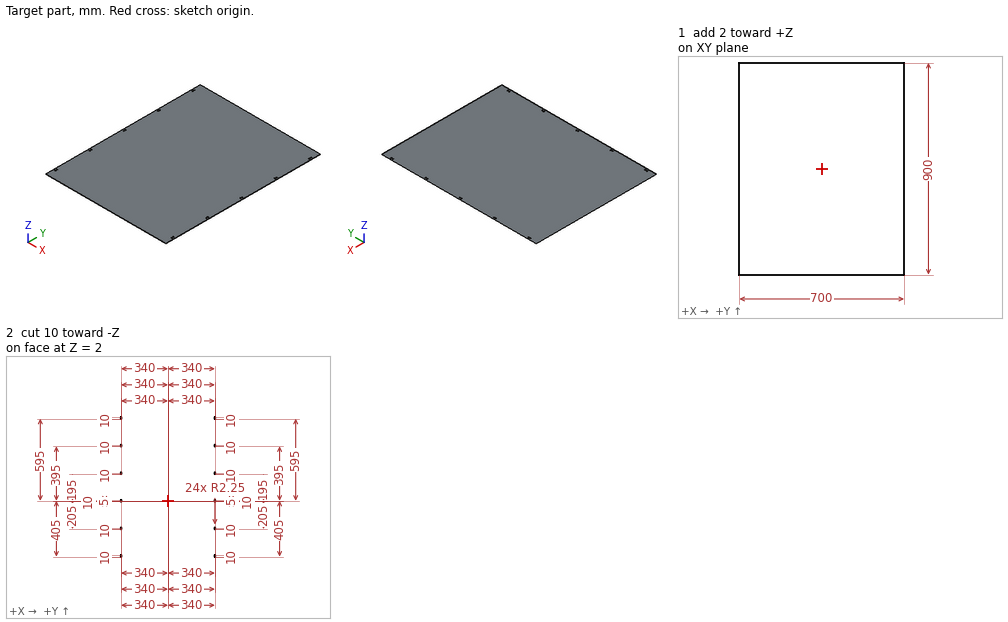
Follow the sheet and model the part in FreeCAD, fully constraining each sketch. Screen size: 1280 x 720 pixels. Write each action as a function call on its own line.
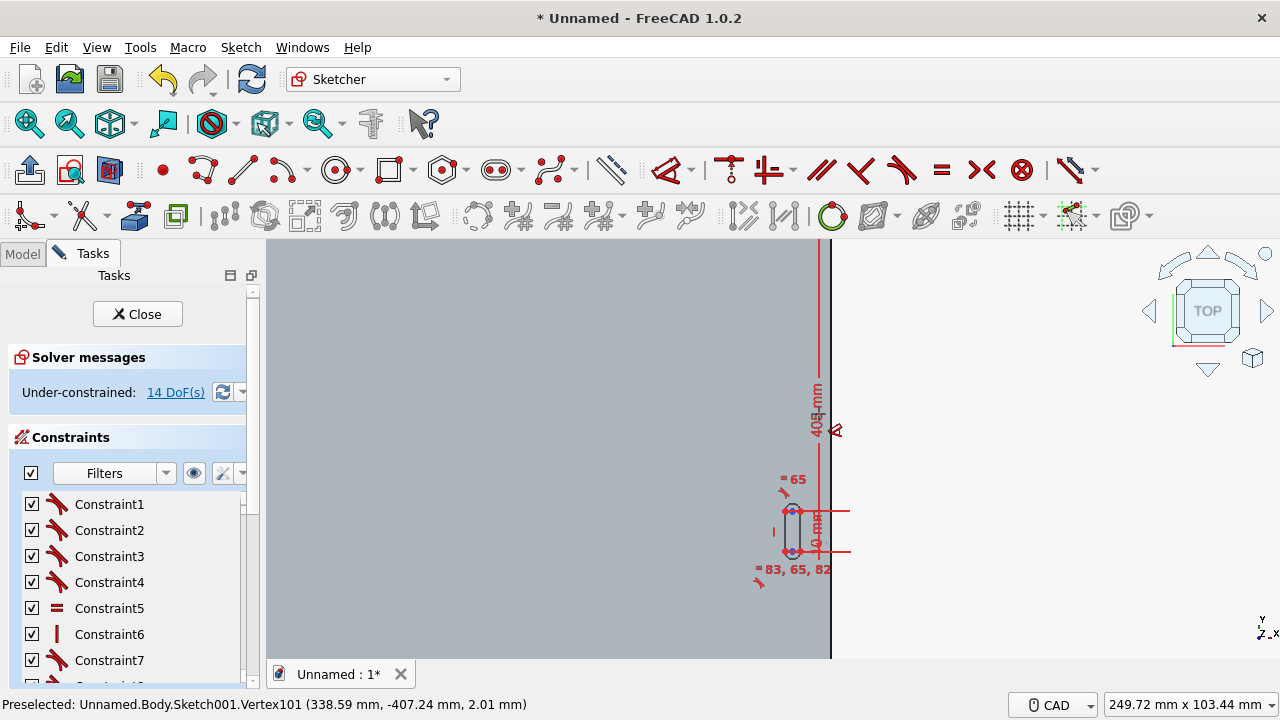
scroll(788, 575, down, 14)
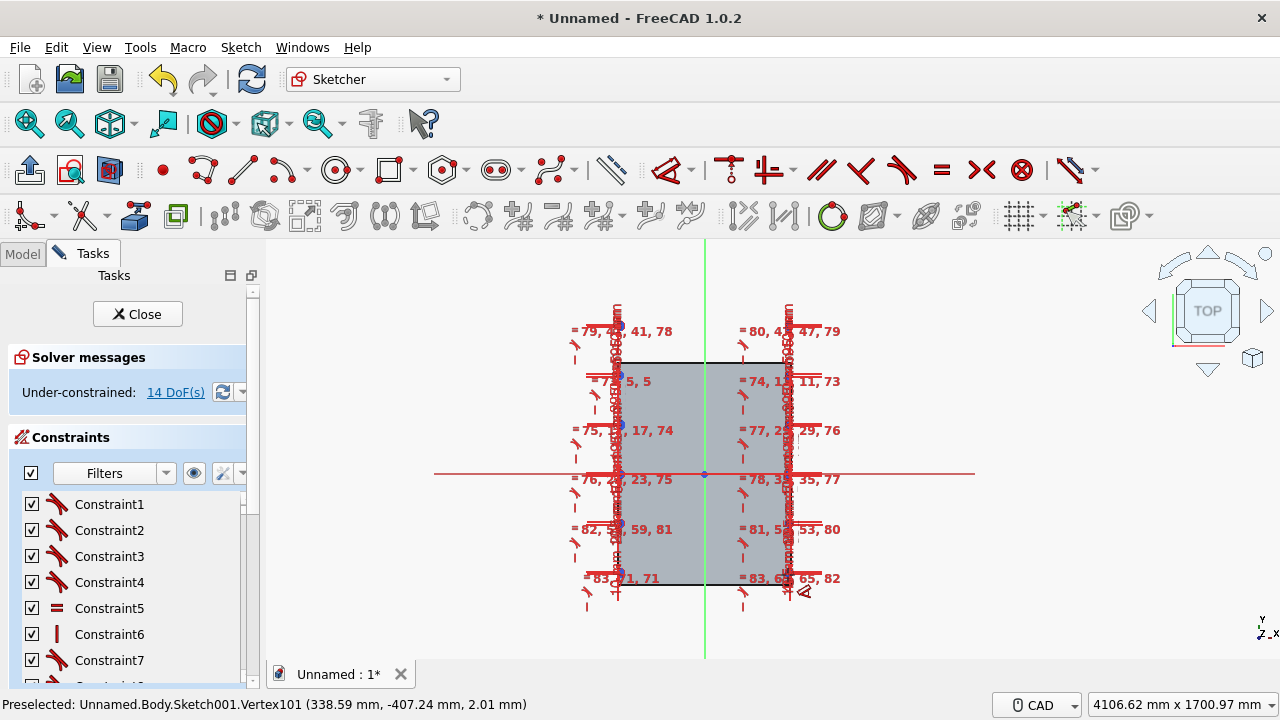
scroll(620, 574, up, 14)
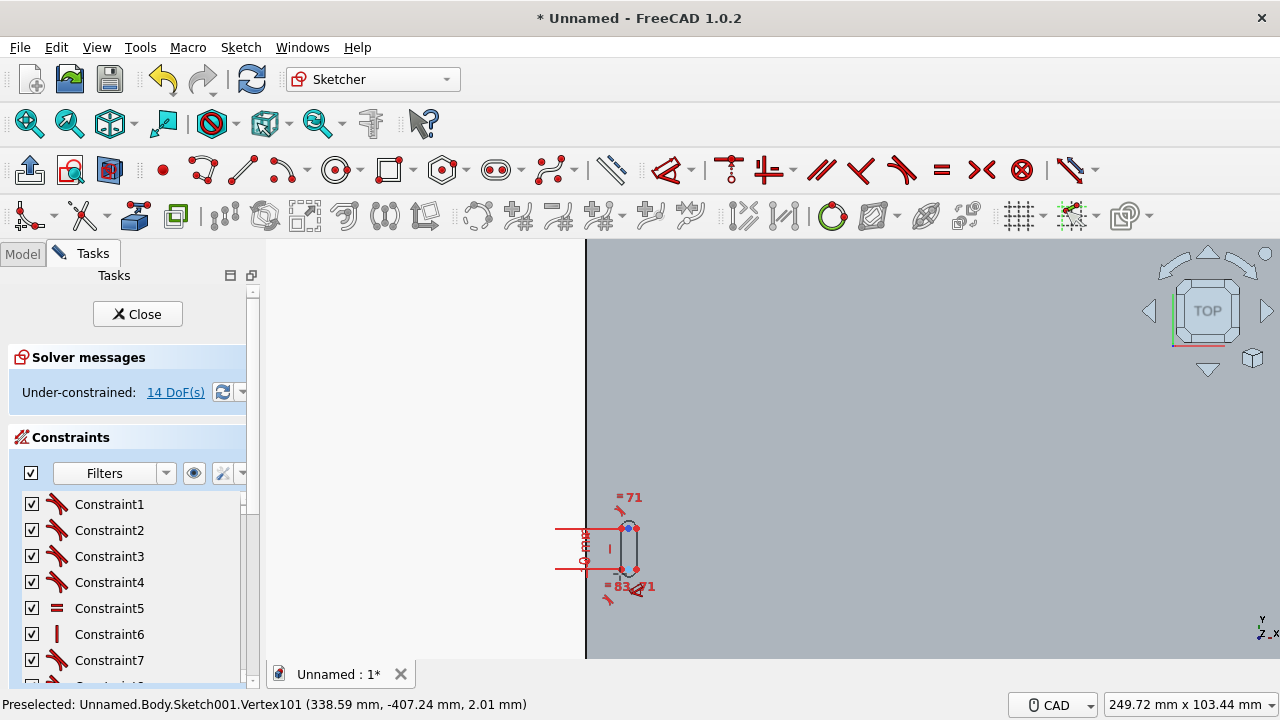
click(621, 569)
click(587, 418)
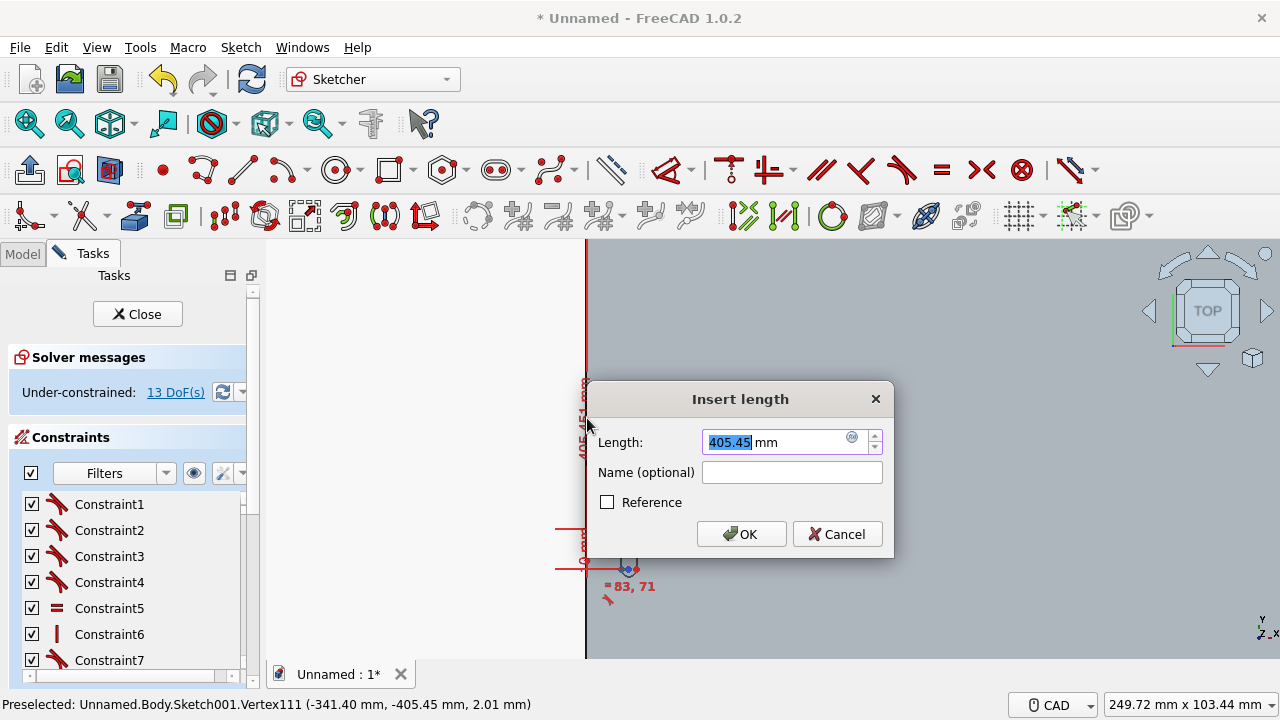
text(405)
key(Return)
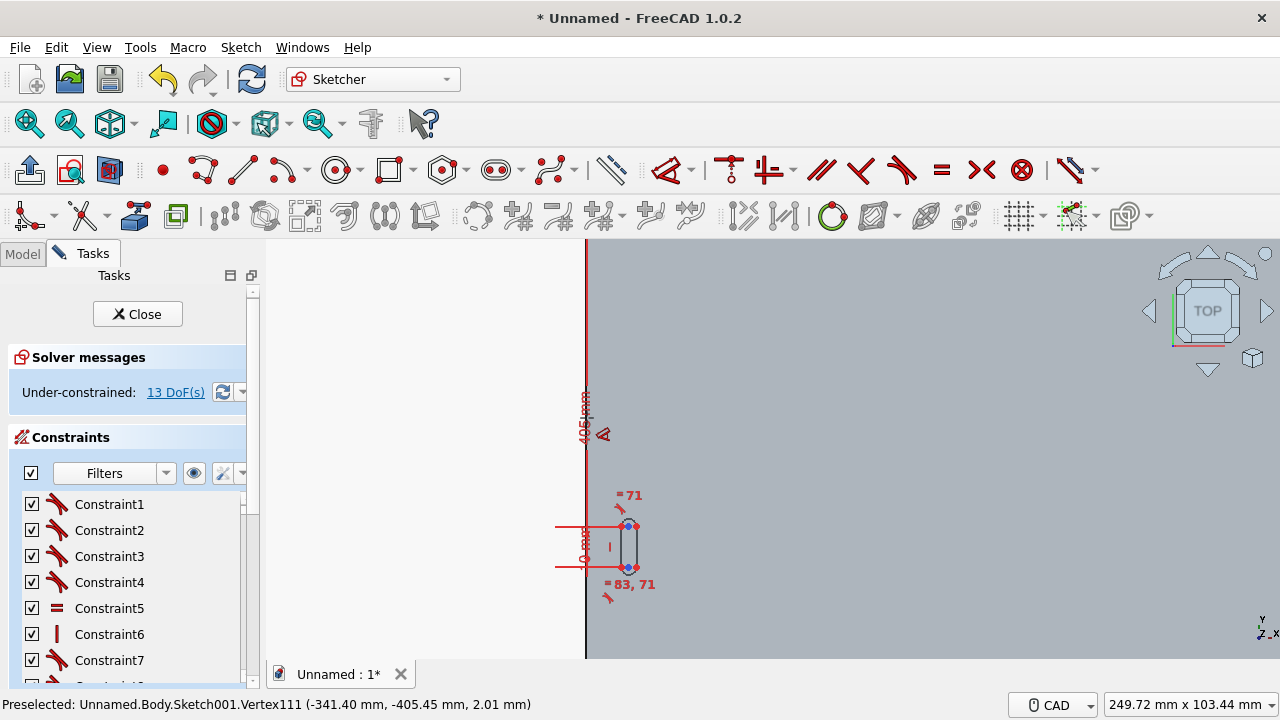
scroll(620, 574, down, 14)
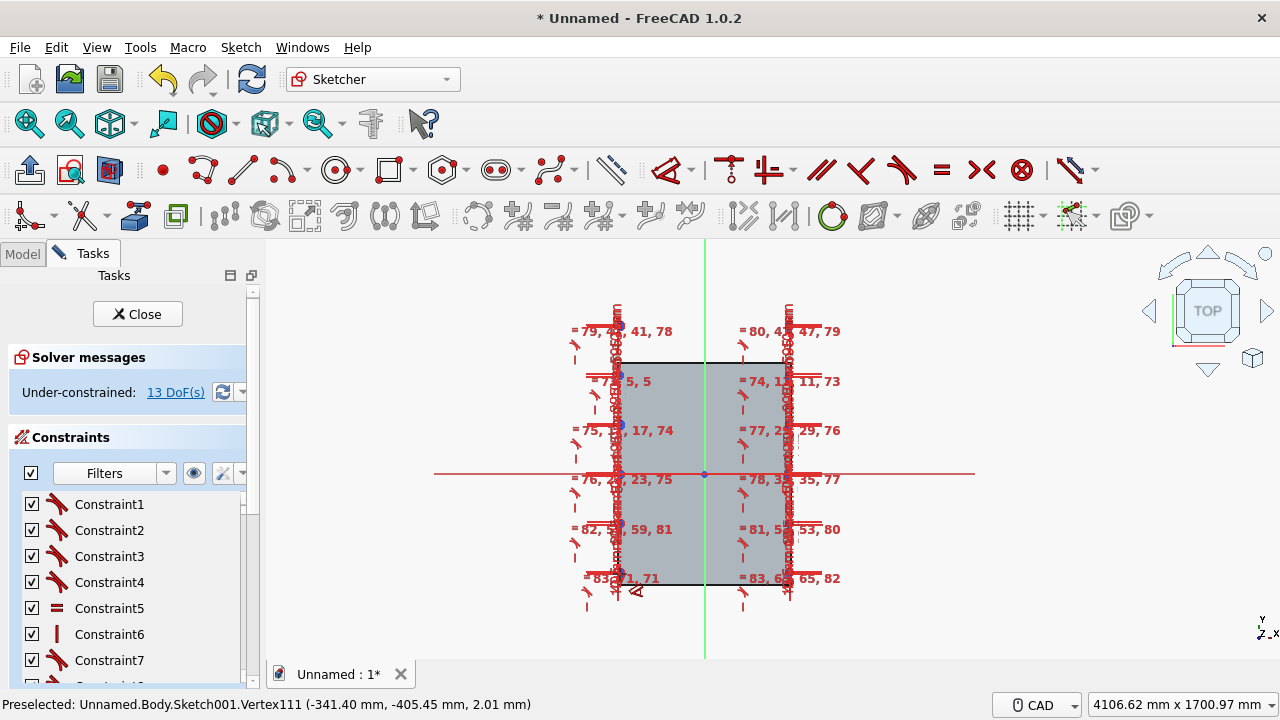
scroll(620, 377, up, 14)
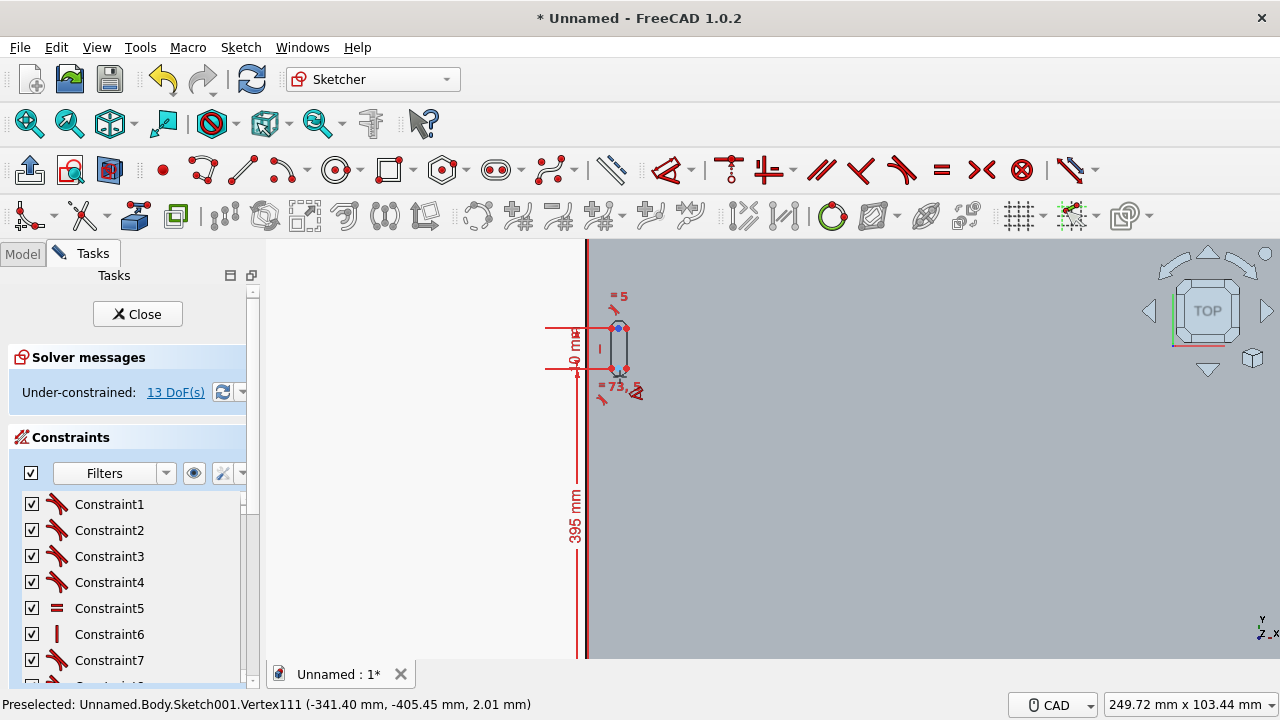
click(619, 369)
click(867, 335)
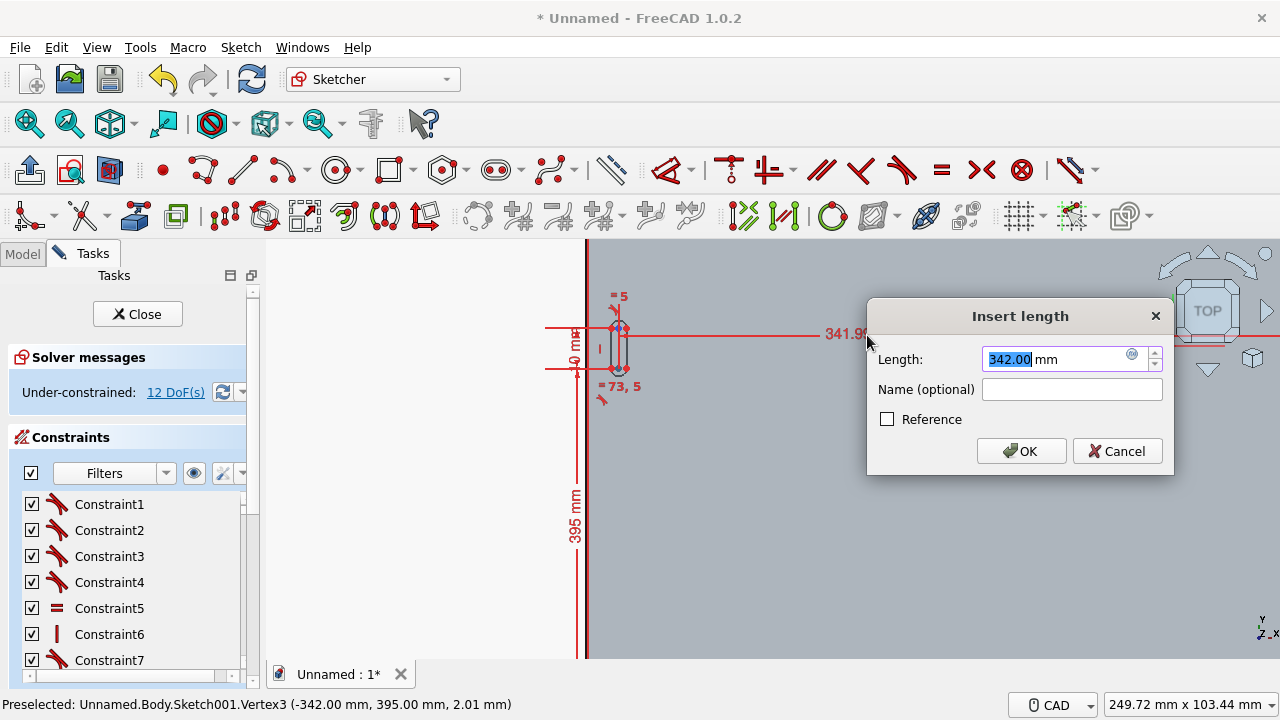
text(340)
key(Return)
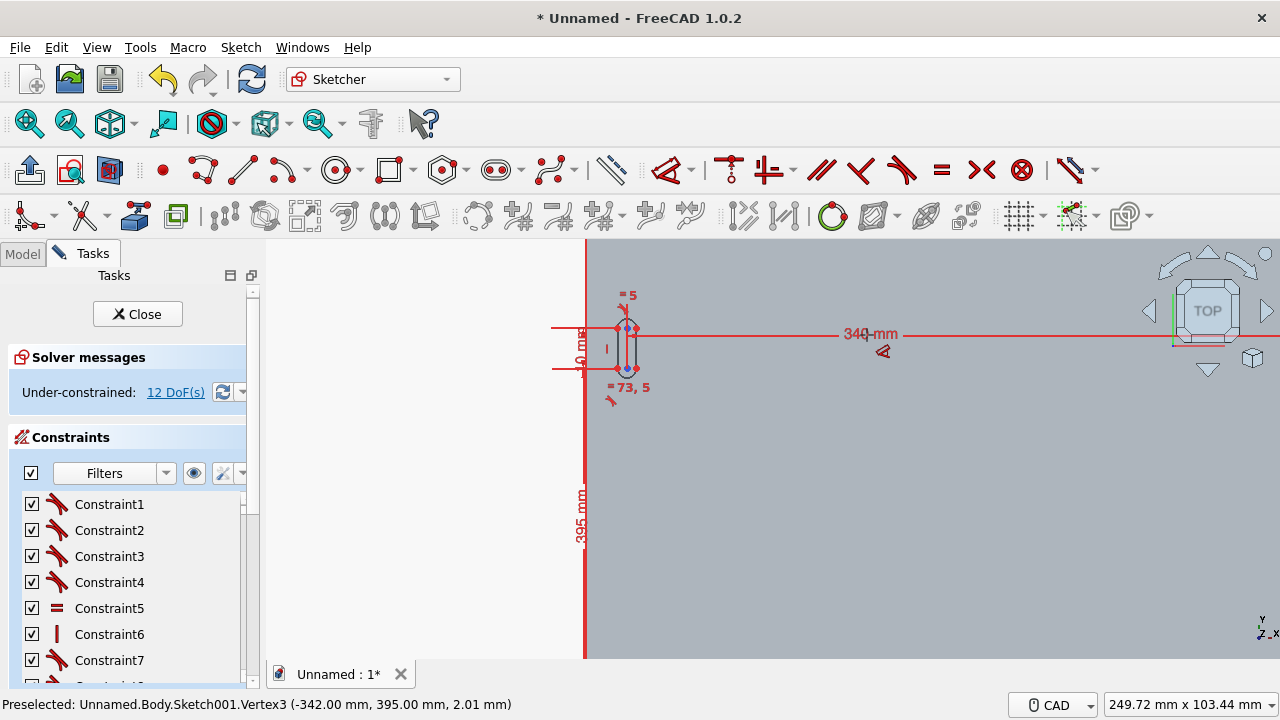
scroll(620, 377, down, 14)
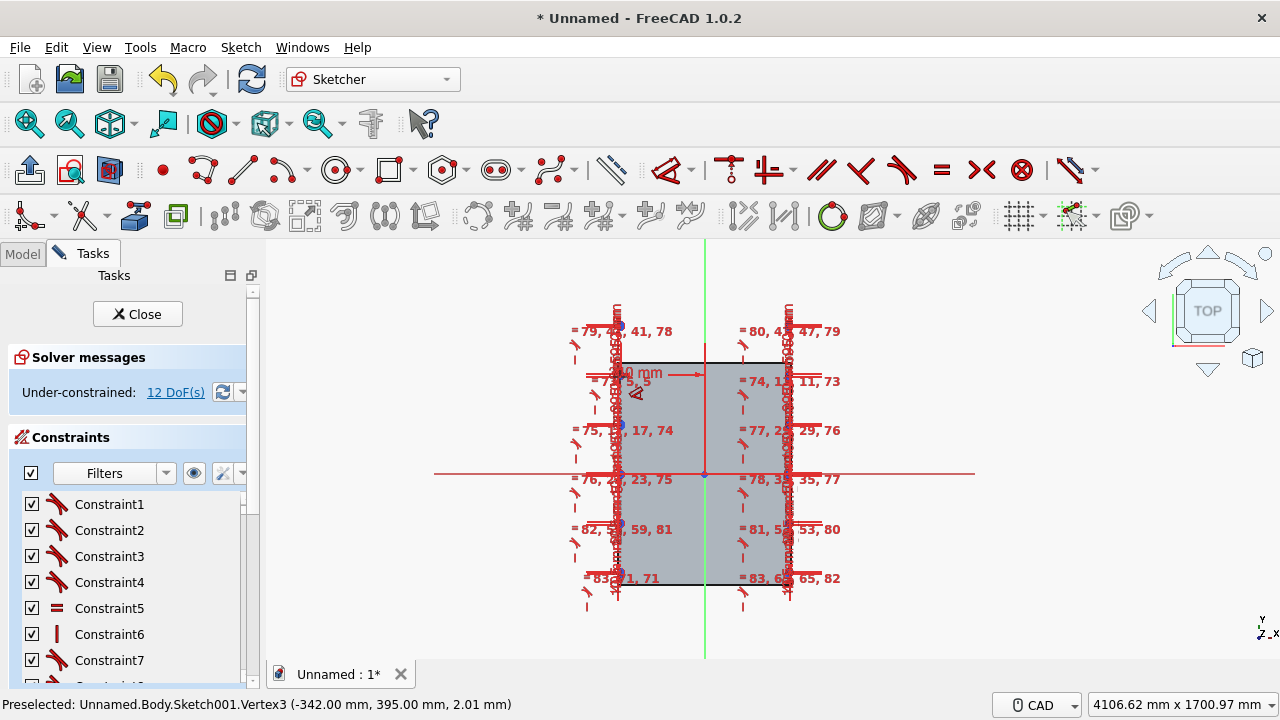
scroll(789, 377, up, 14)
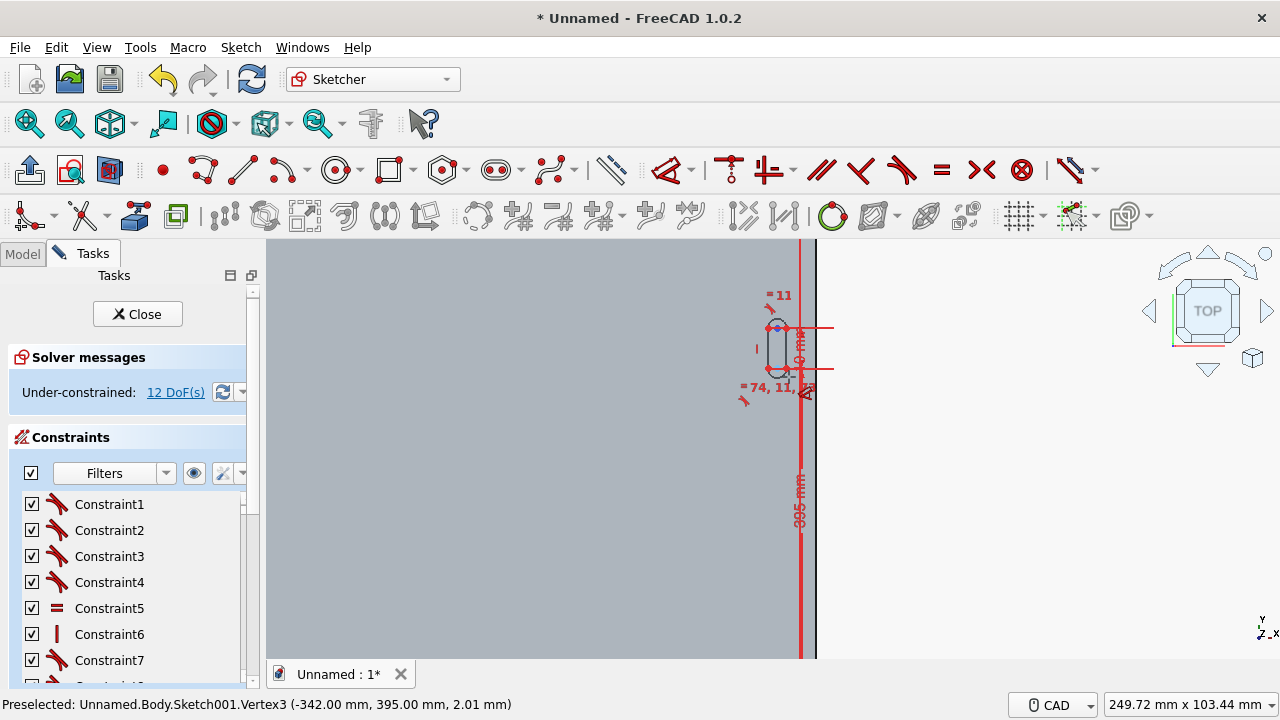
click(777, 369)
click(536, 335)